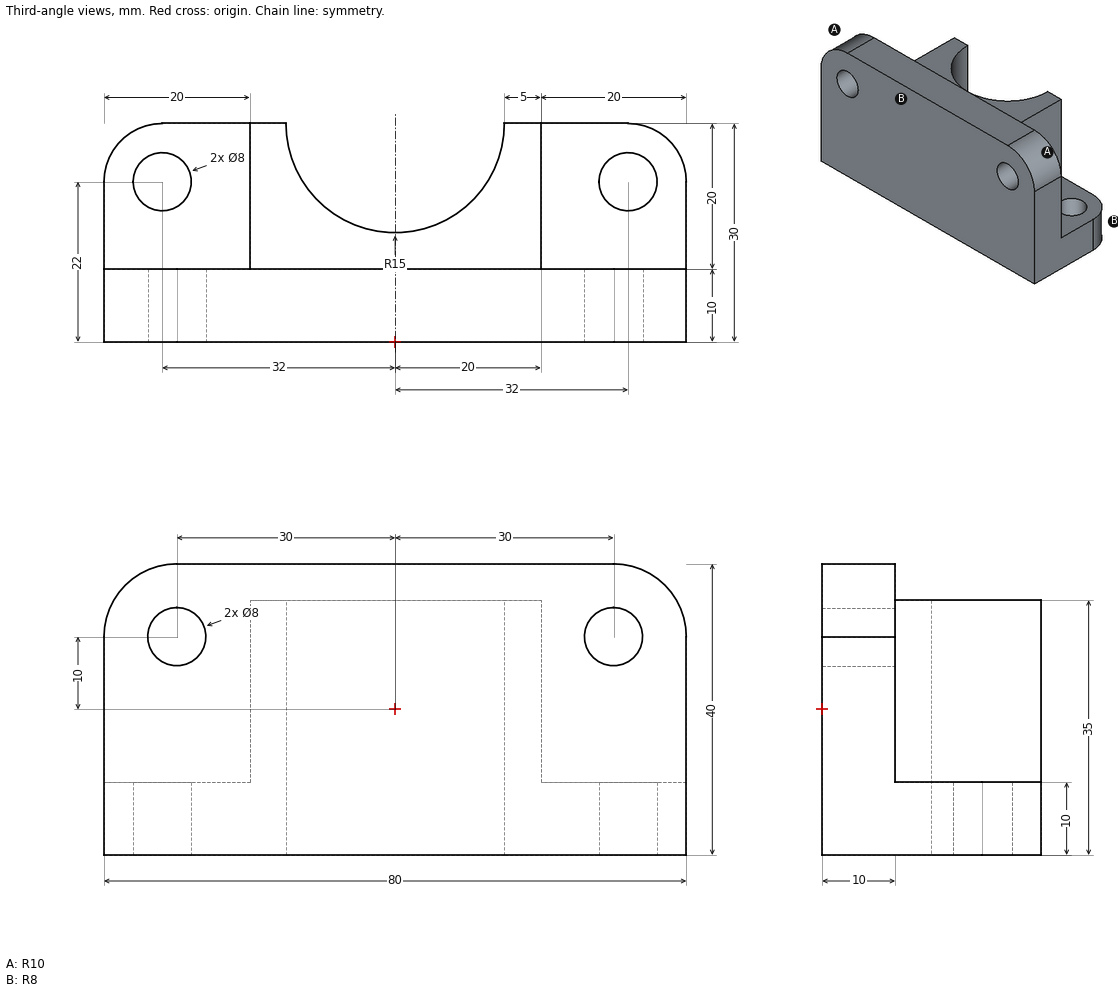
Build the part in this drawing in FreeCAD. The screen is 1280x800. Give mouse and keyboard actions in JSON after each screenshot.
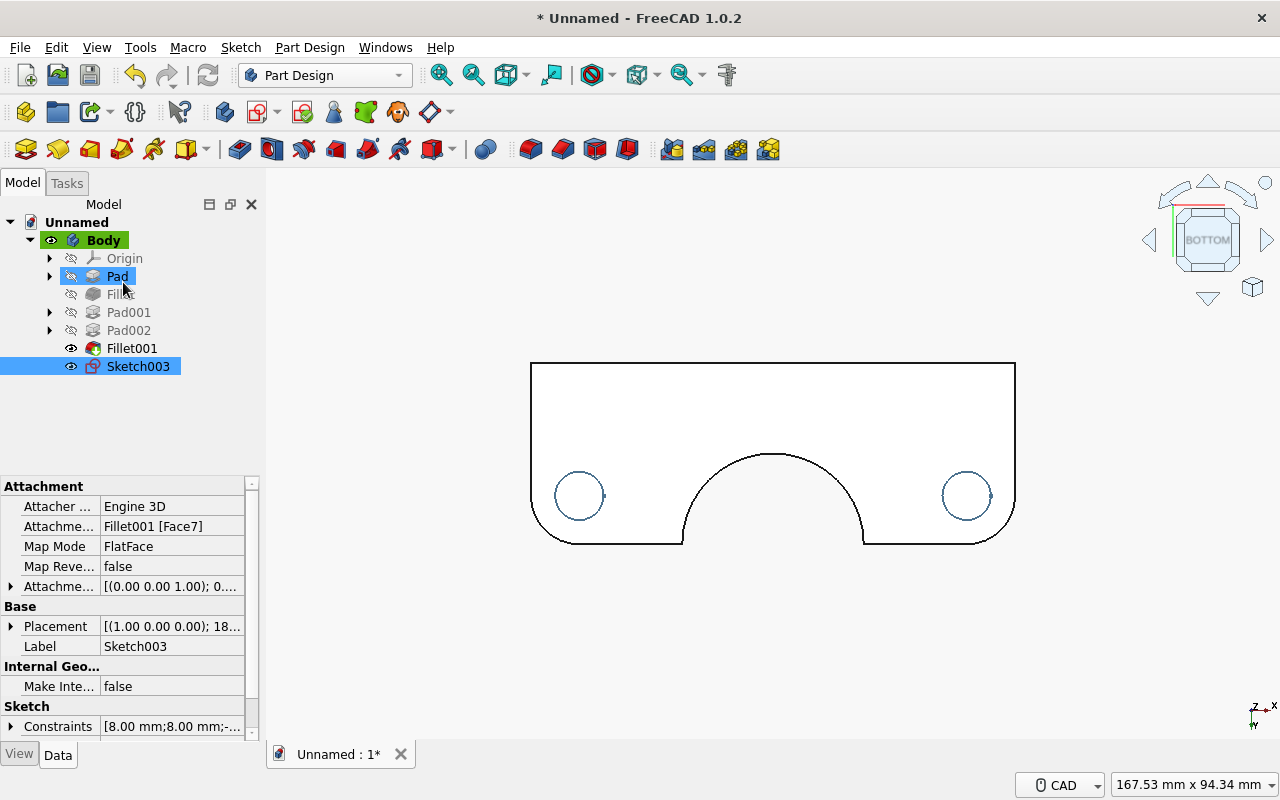
{"action": "left_click", "coordinate": [240, 150]}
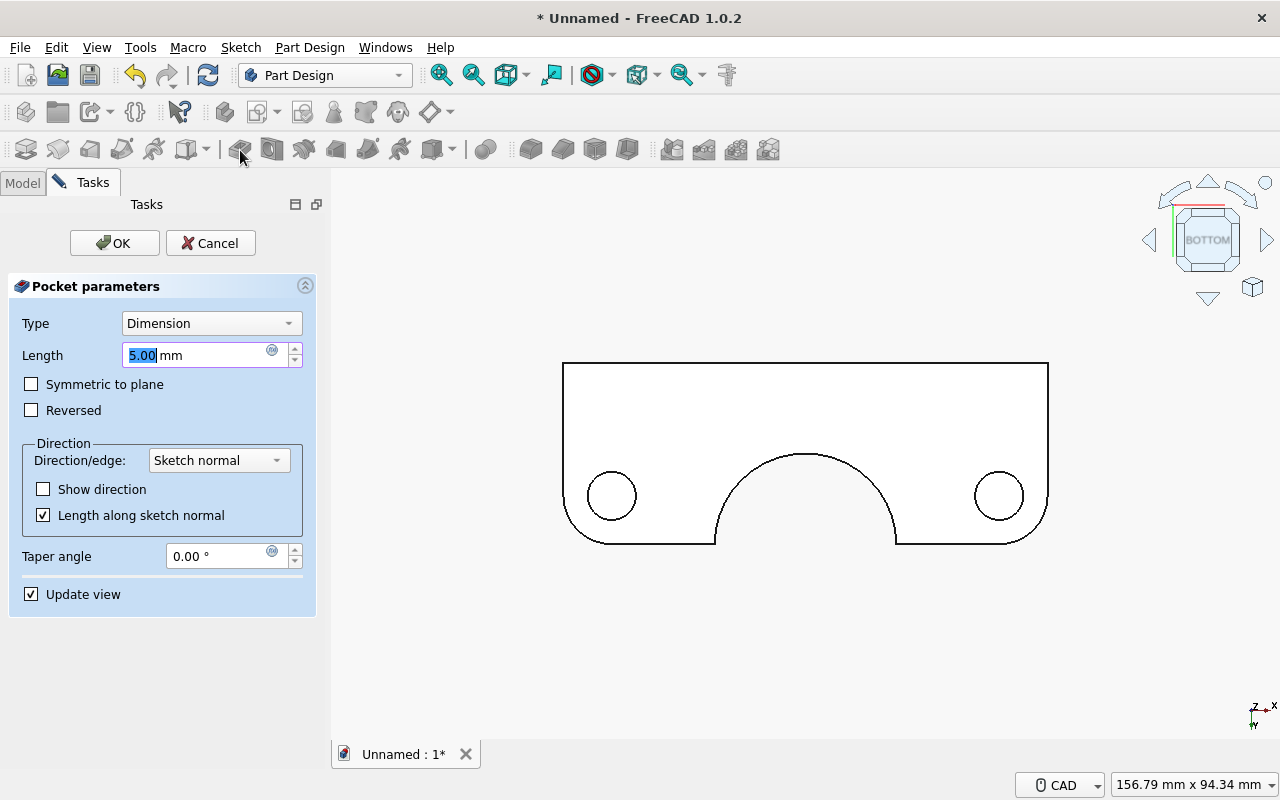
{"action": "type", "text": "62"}
{"action": "key", "text": "Tab"}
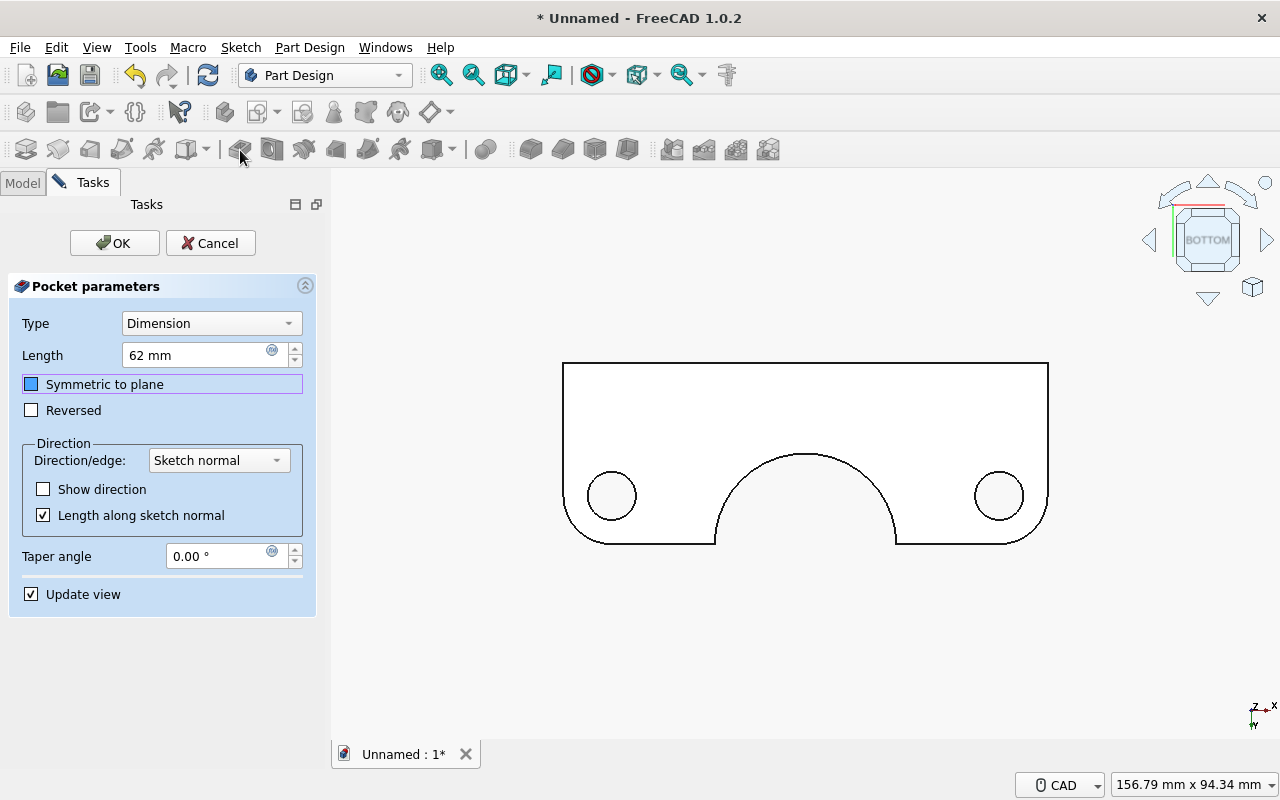
{"action": "left_click", "coordinate": [115, 243]}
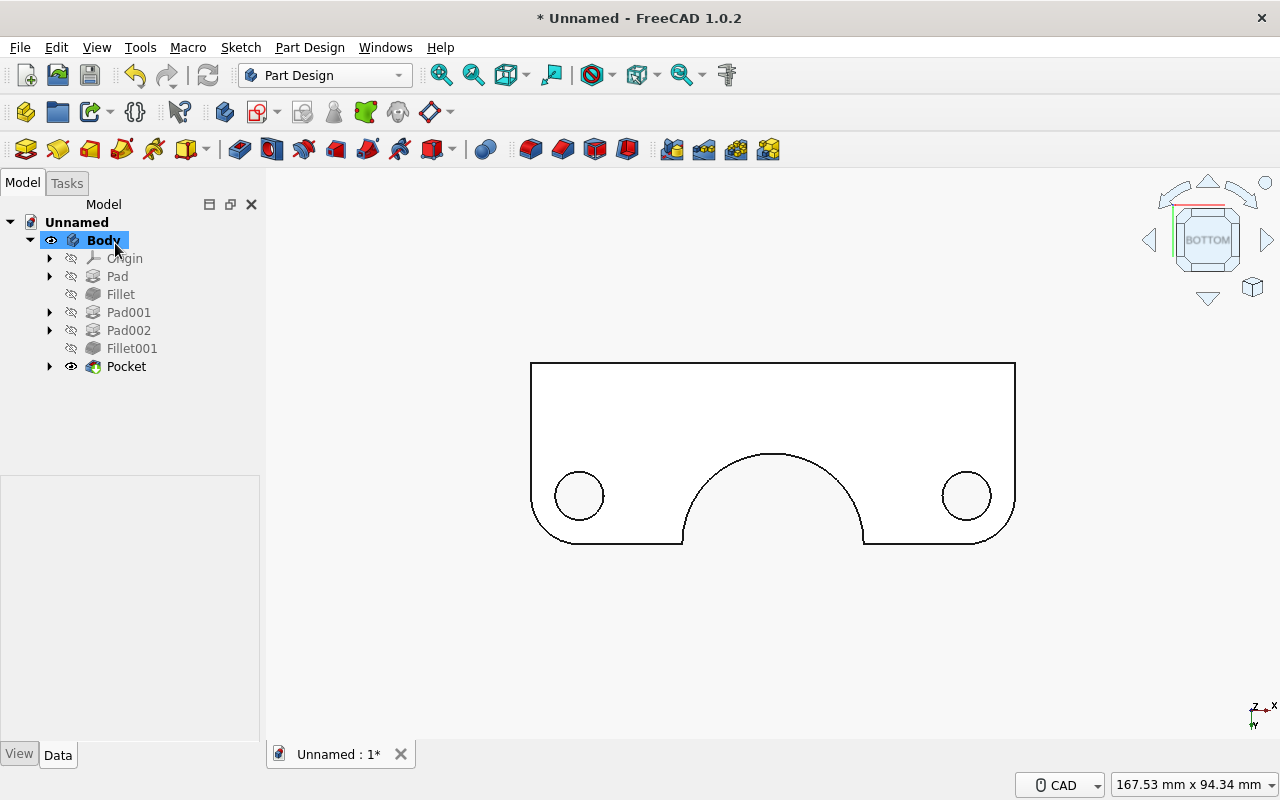
{"action": "key", "text": "4"}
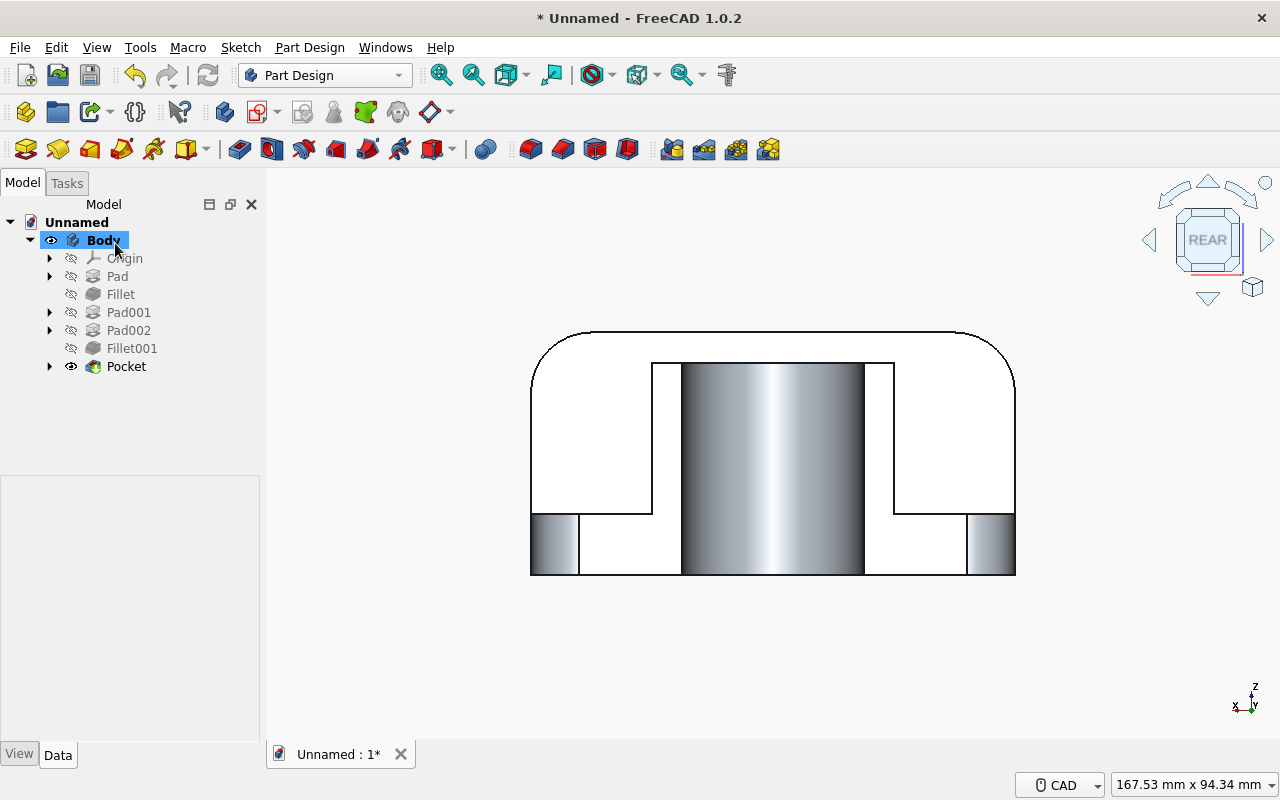
{"action": "left_click", "coordinate": [981, 396]}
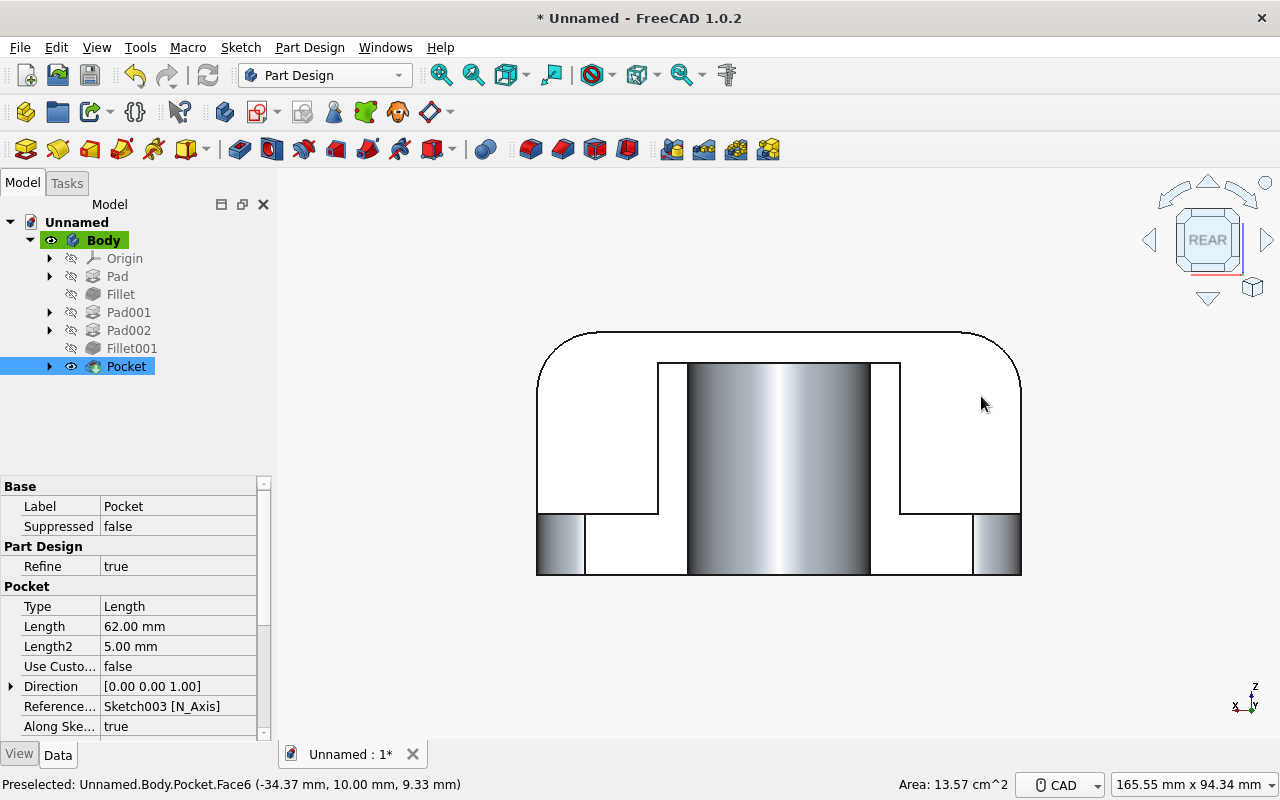
{"action": "left_click", "coordinate": [258, 112]}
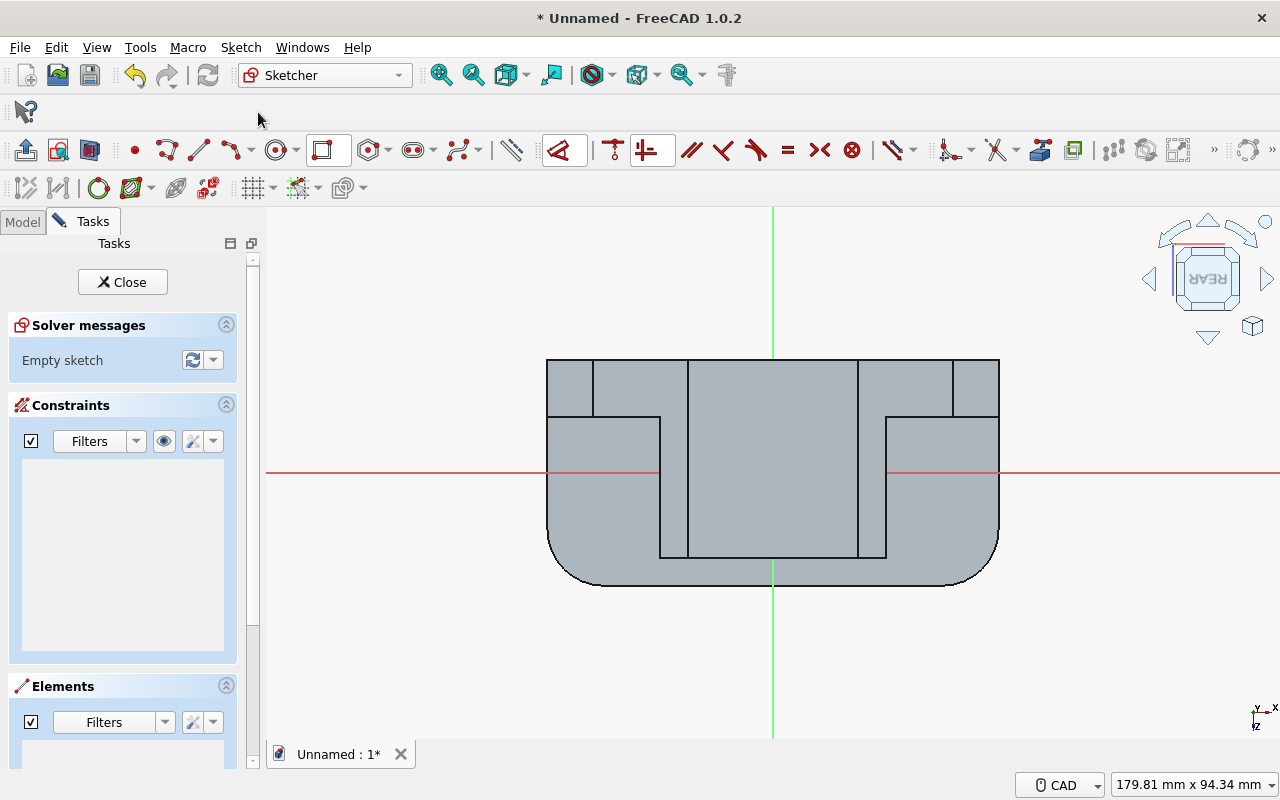
{"action": "scroll", "coordinate": [912, 593], "scroll_direction": "up", "scroll_amount": 2}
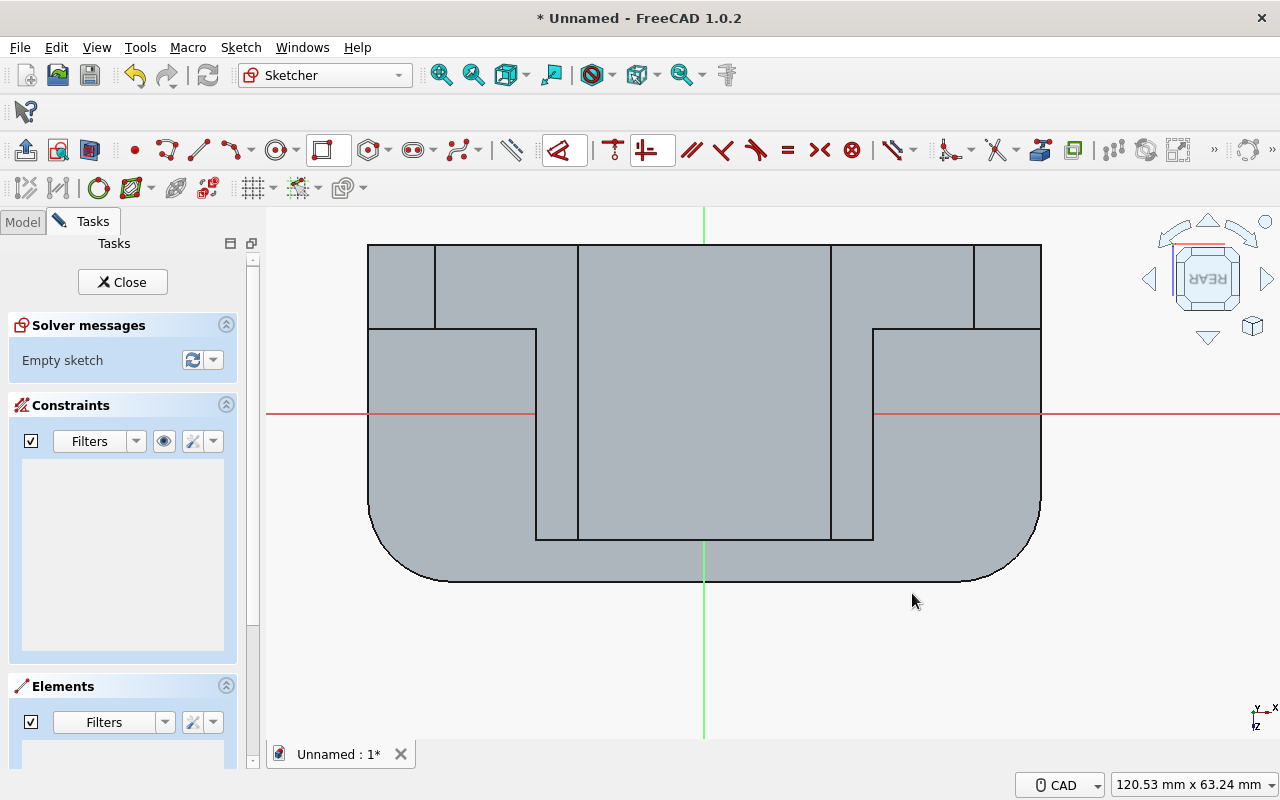
{"action": "left_click", "coordinate": [276, 150]}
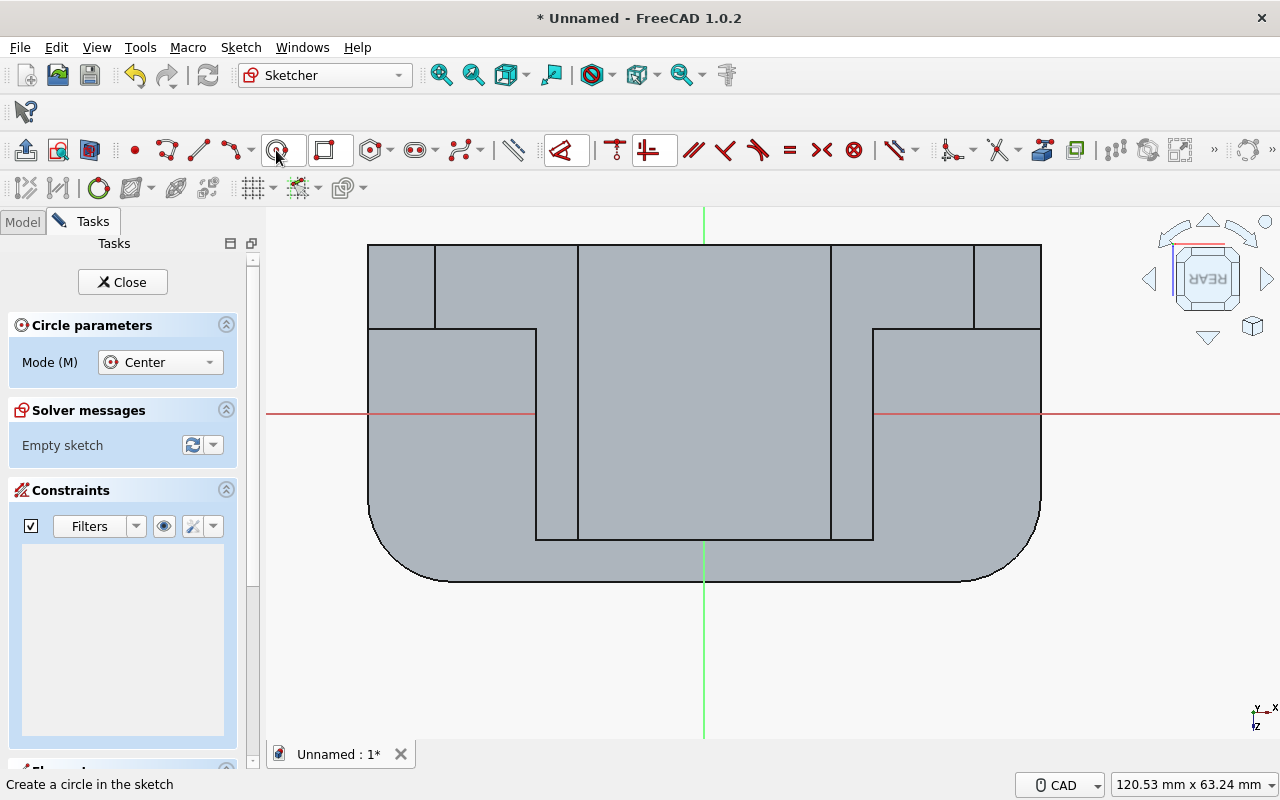
{"action": "left_click", "coordinate": [452, 498]}
{"action": "mouse_move", "coordinate": [476, 474]}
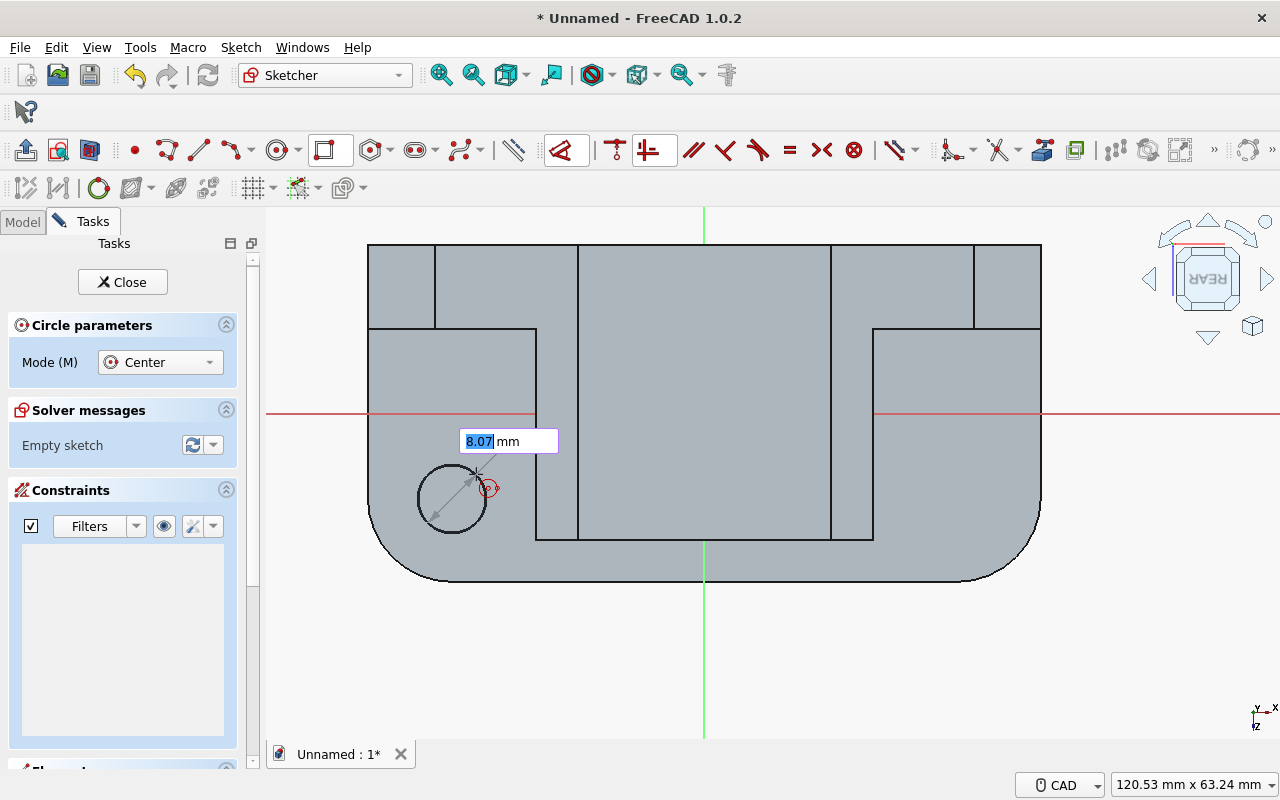
{"action": "type", "text": "8"}
{"action": "key", "text": "Return"}